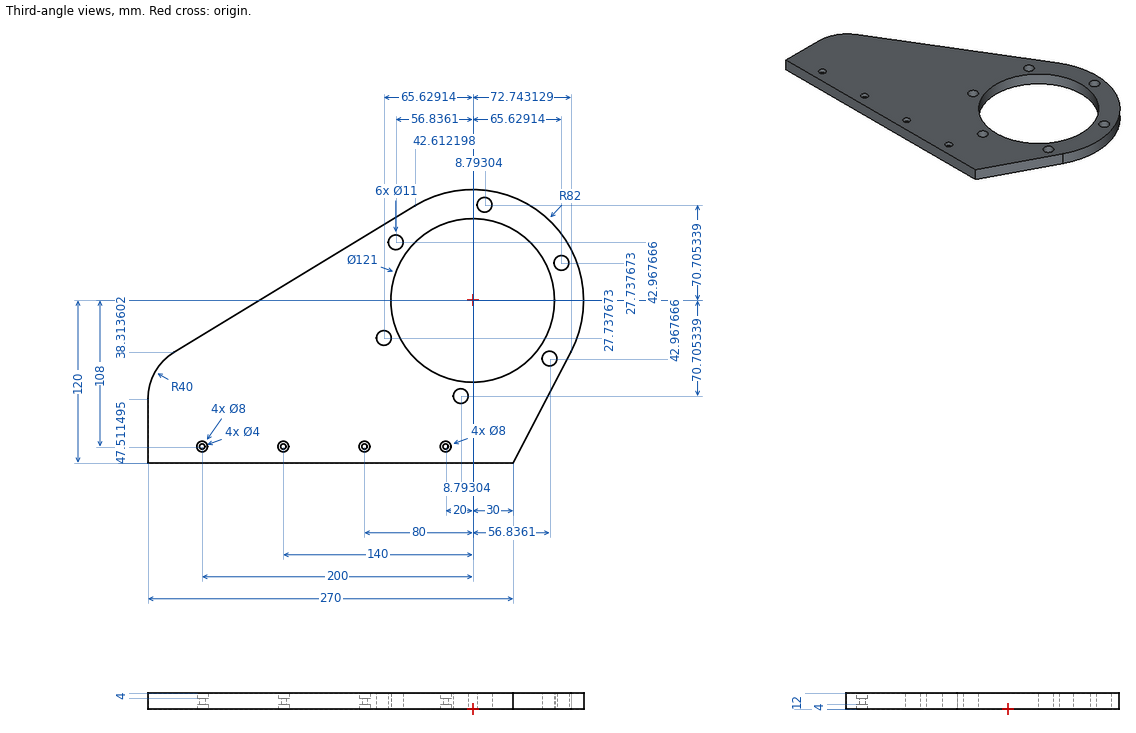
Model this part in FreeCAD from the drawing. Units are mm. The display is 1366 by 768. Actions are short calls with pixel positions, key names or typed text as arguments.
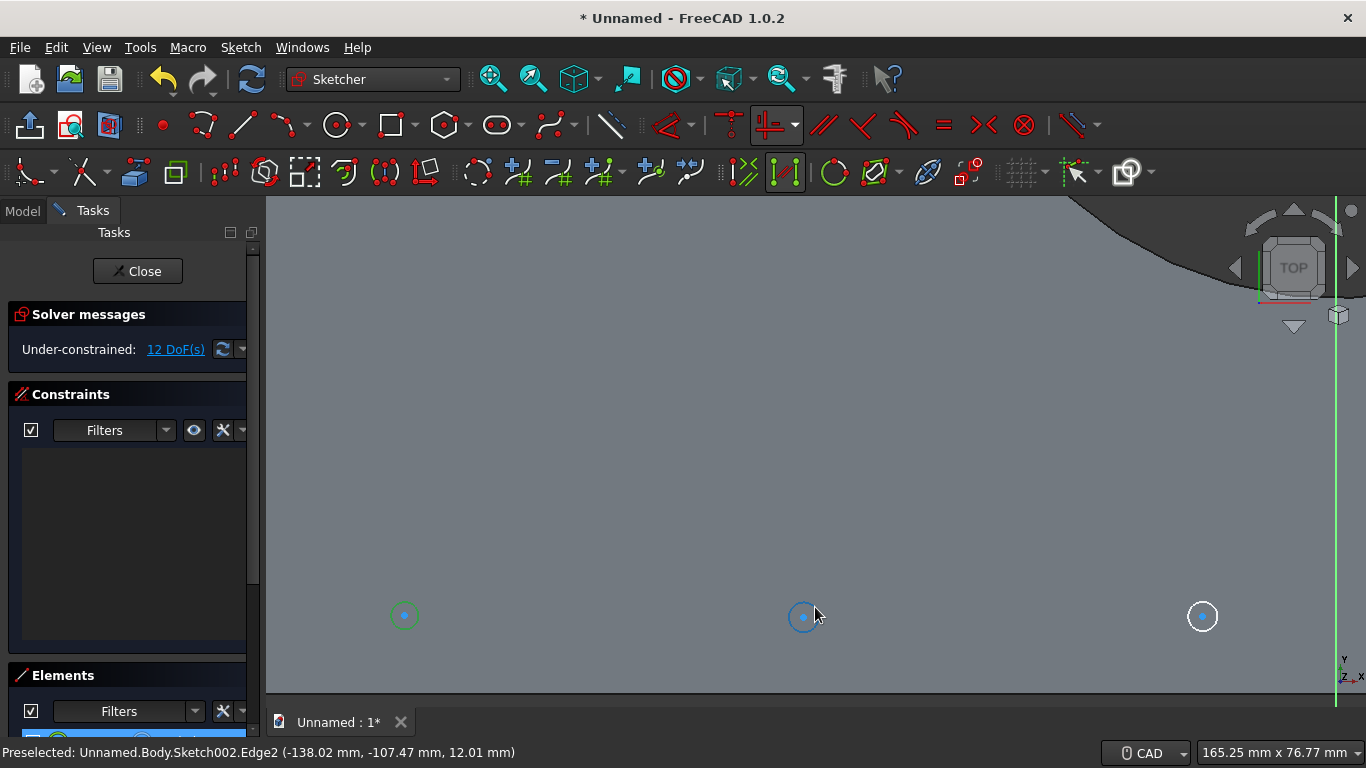
click(814, 607)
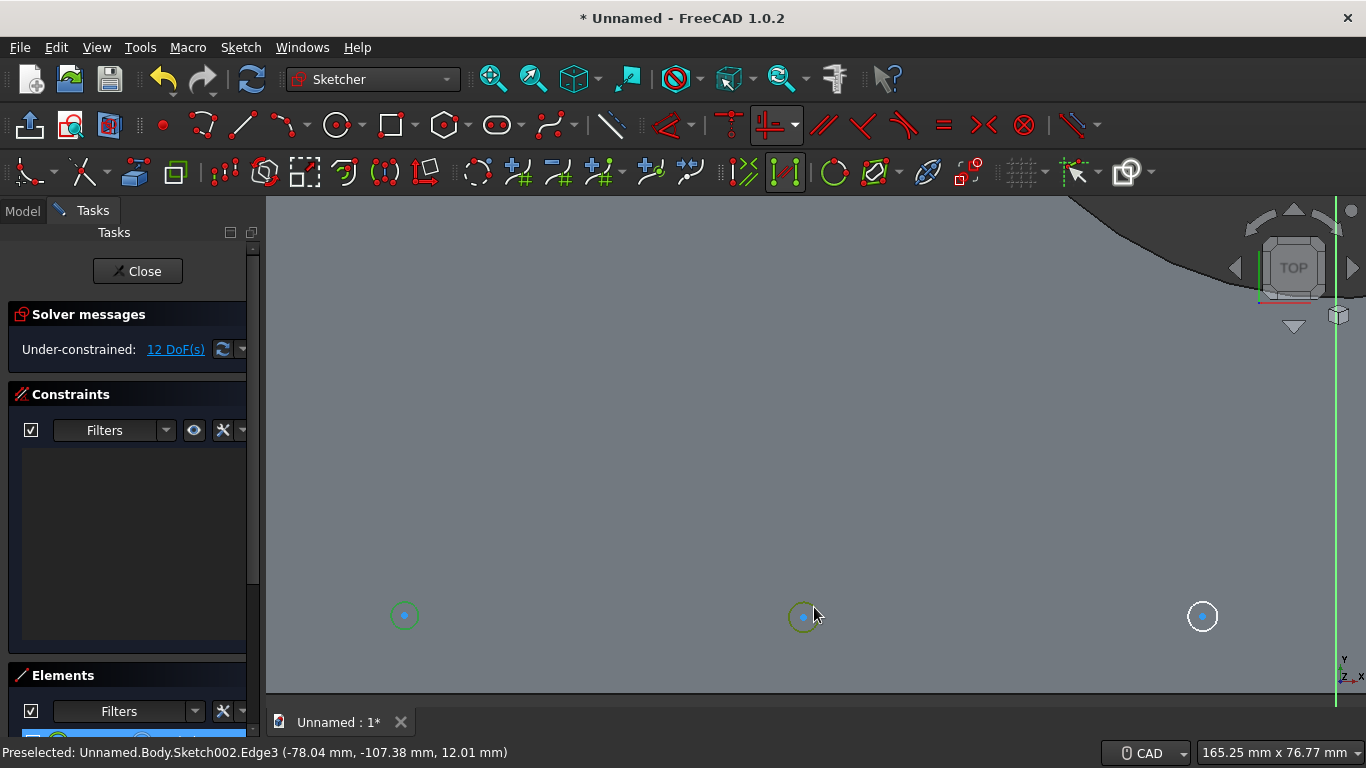
click(1193, 606)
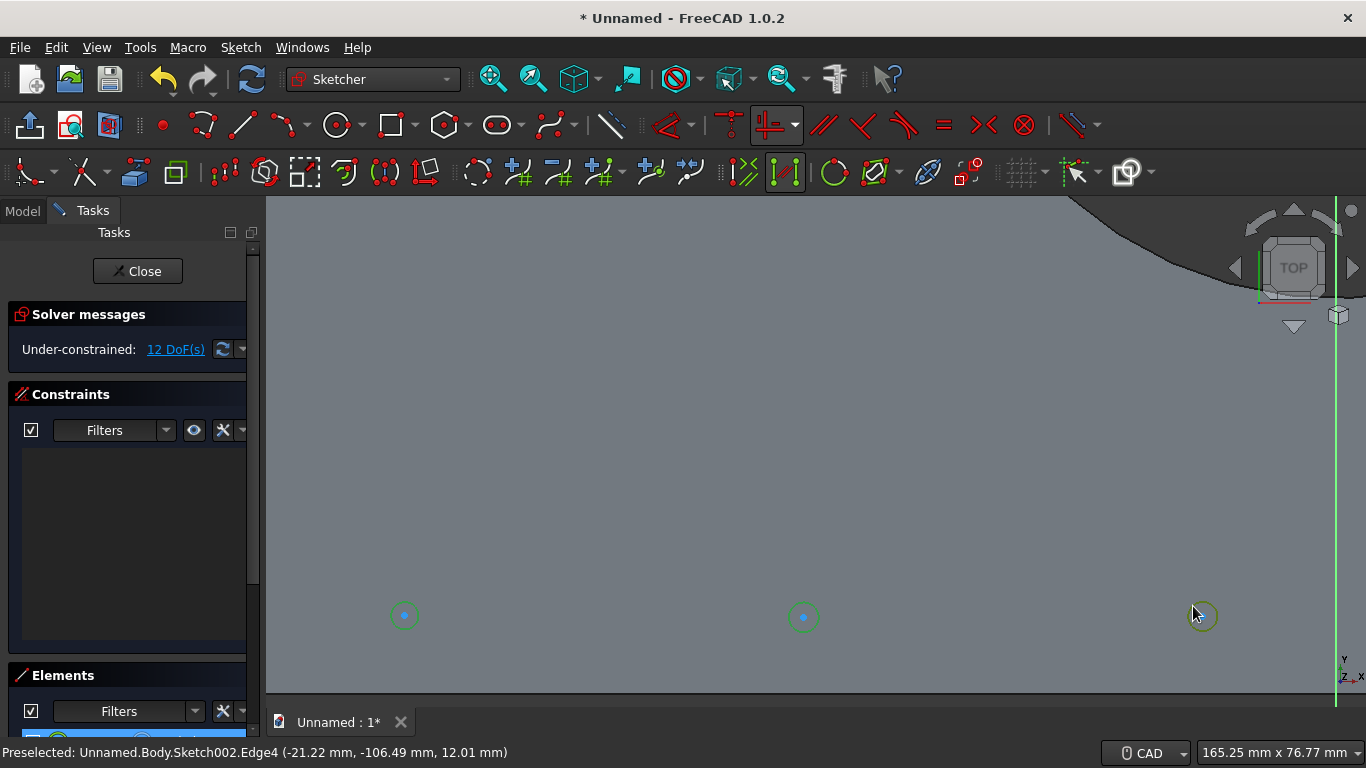
click(944, 126)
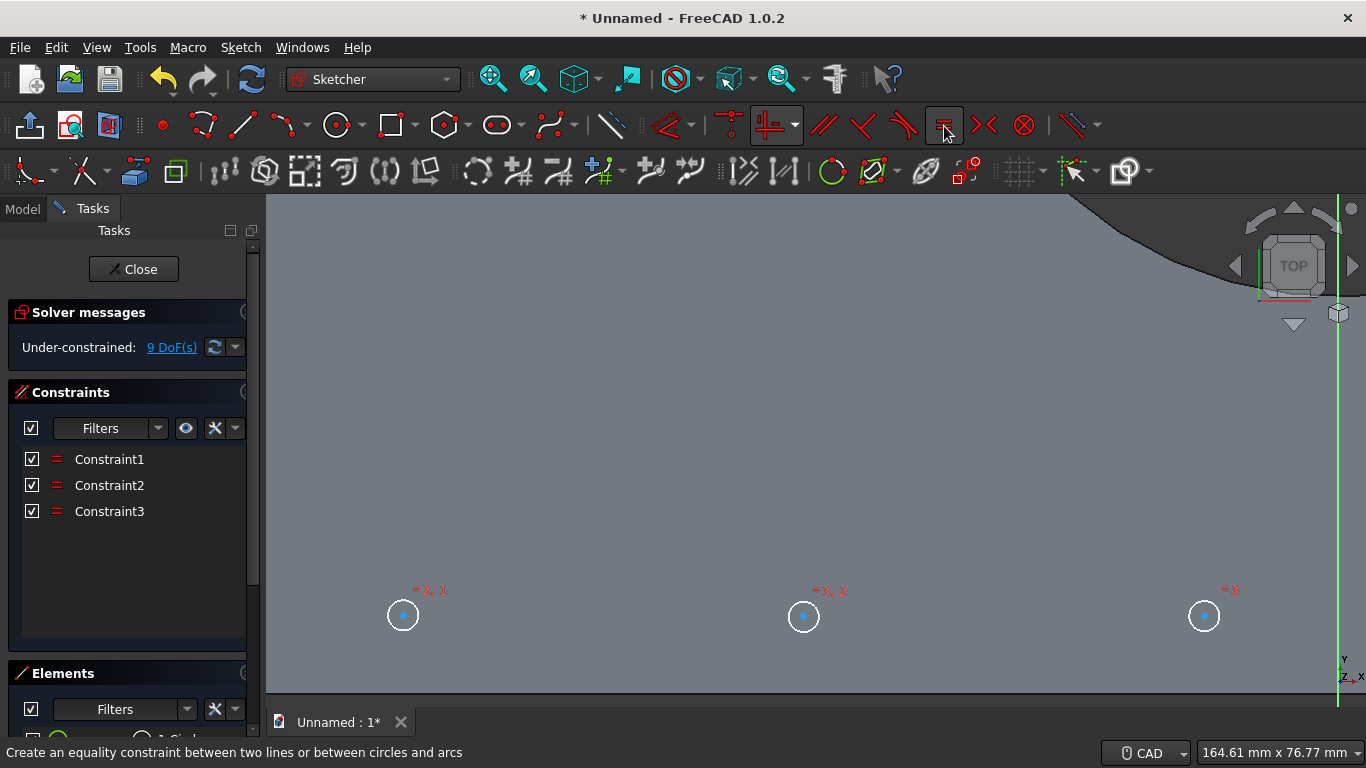
scroll(816, 606, down, 4)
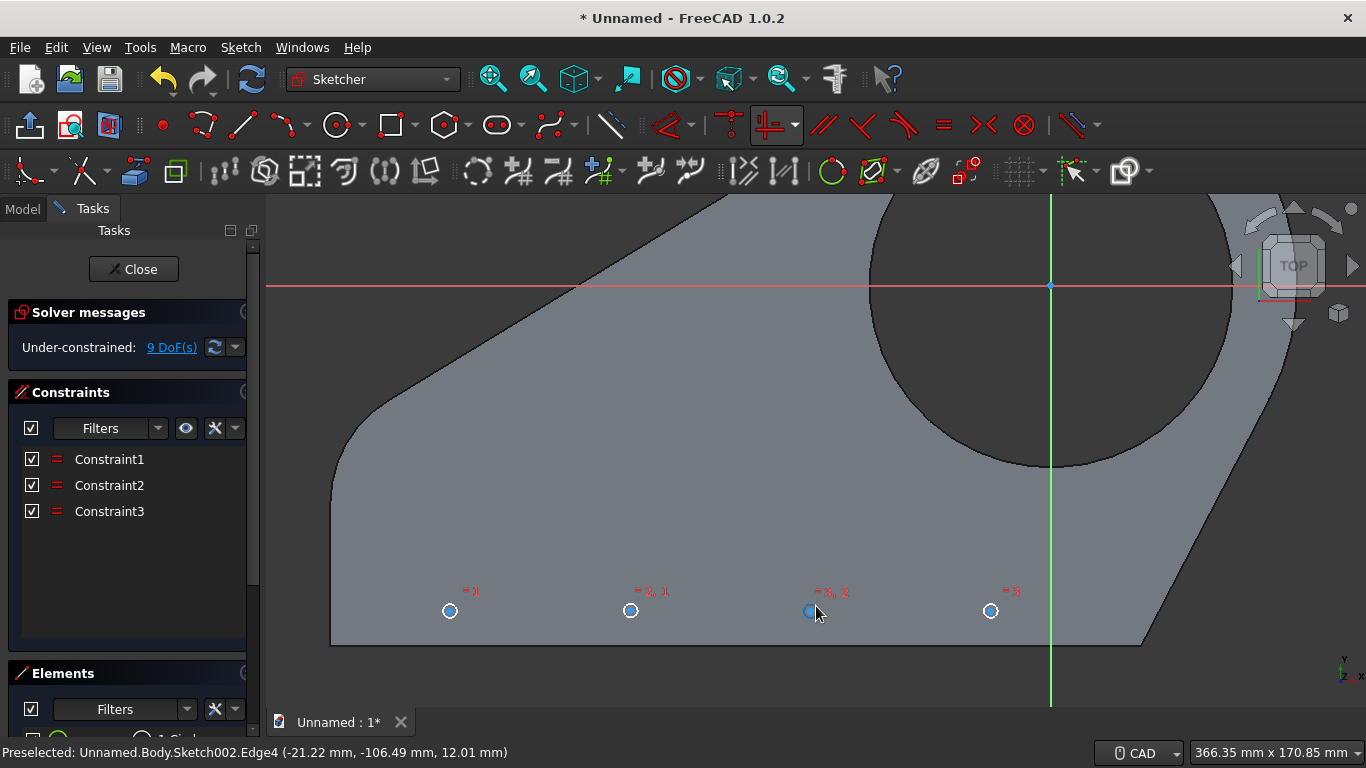
click(450, 611)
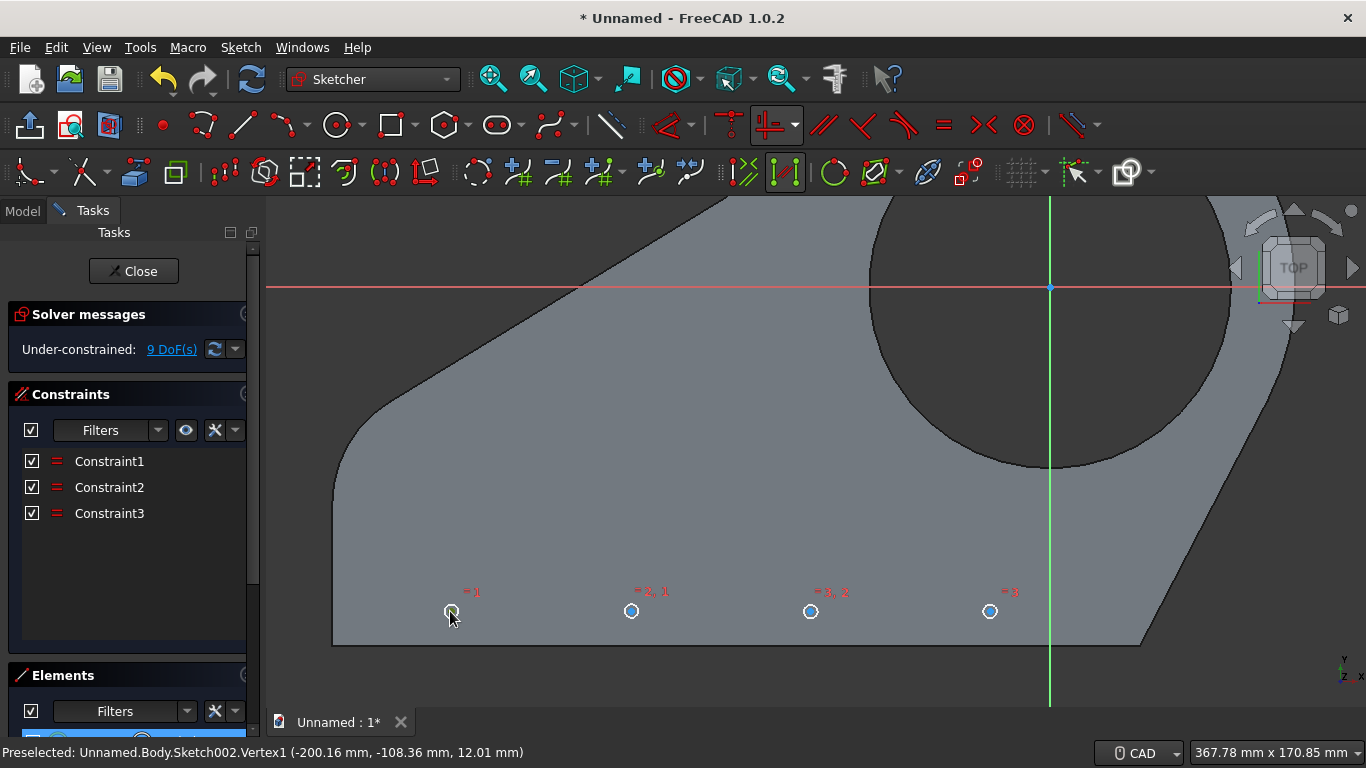
click(632, 611)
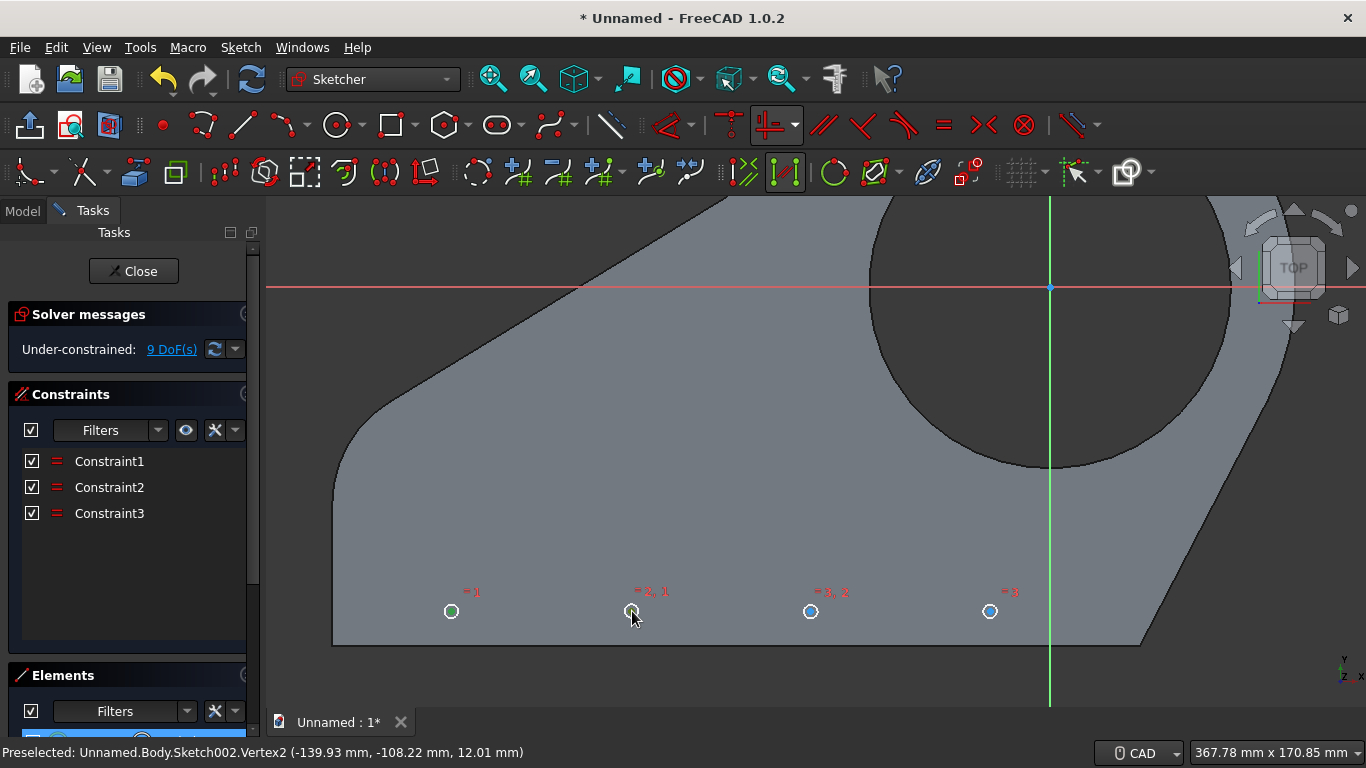
click(798, 126)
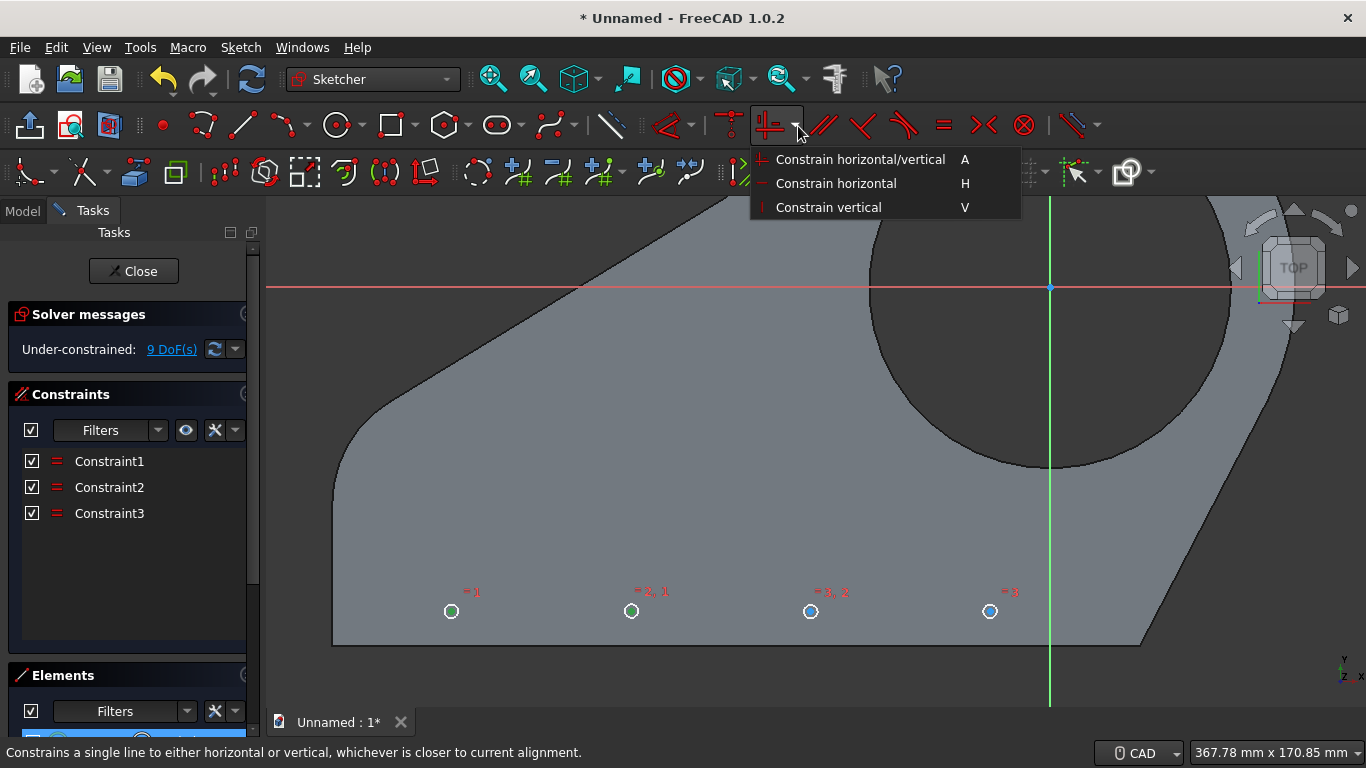
click(886, 183)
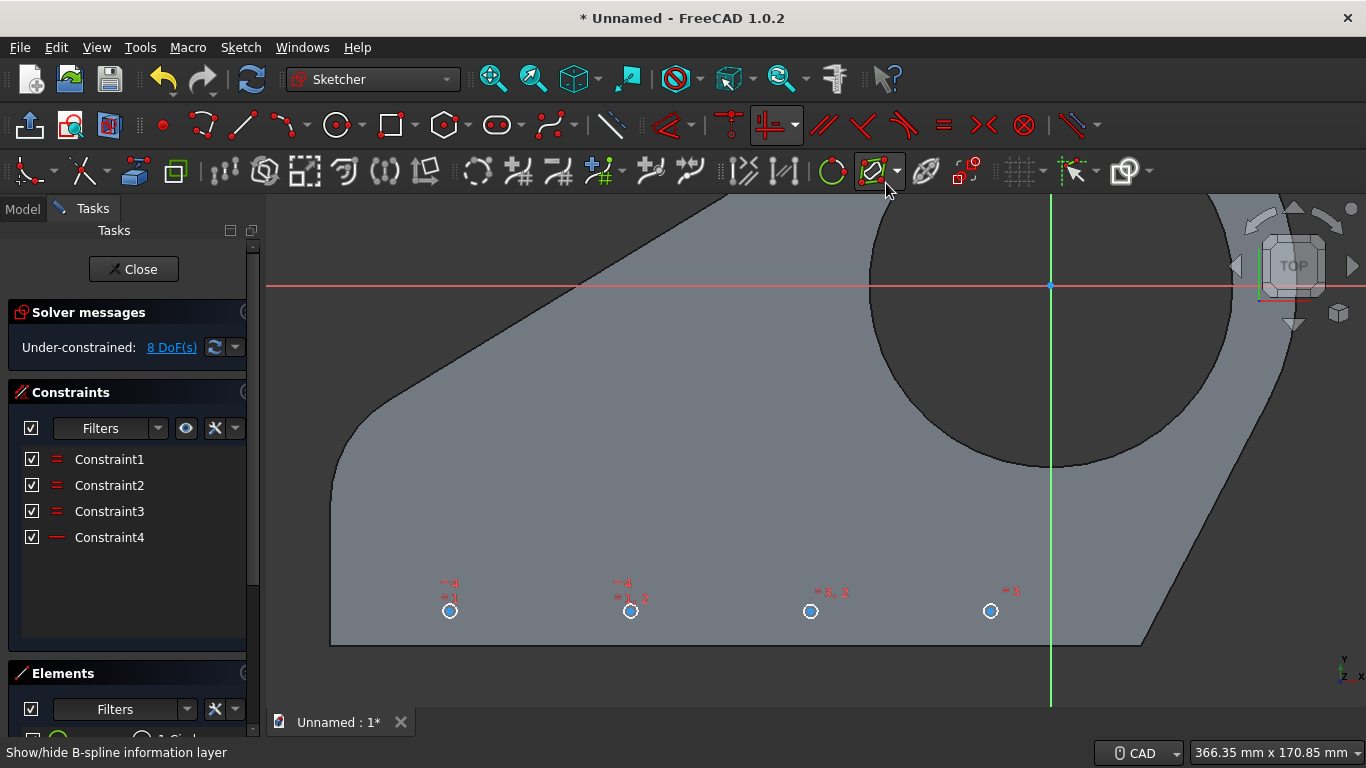
click(631, 611)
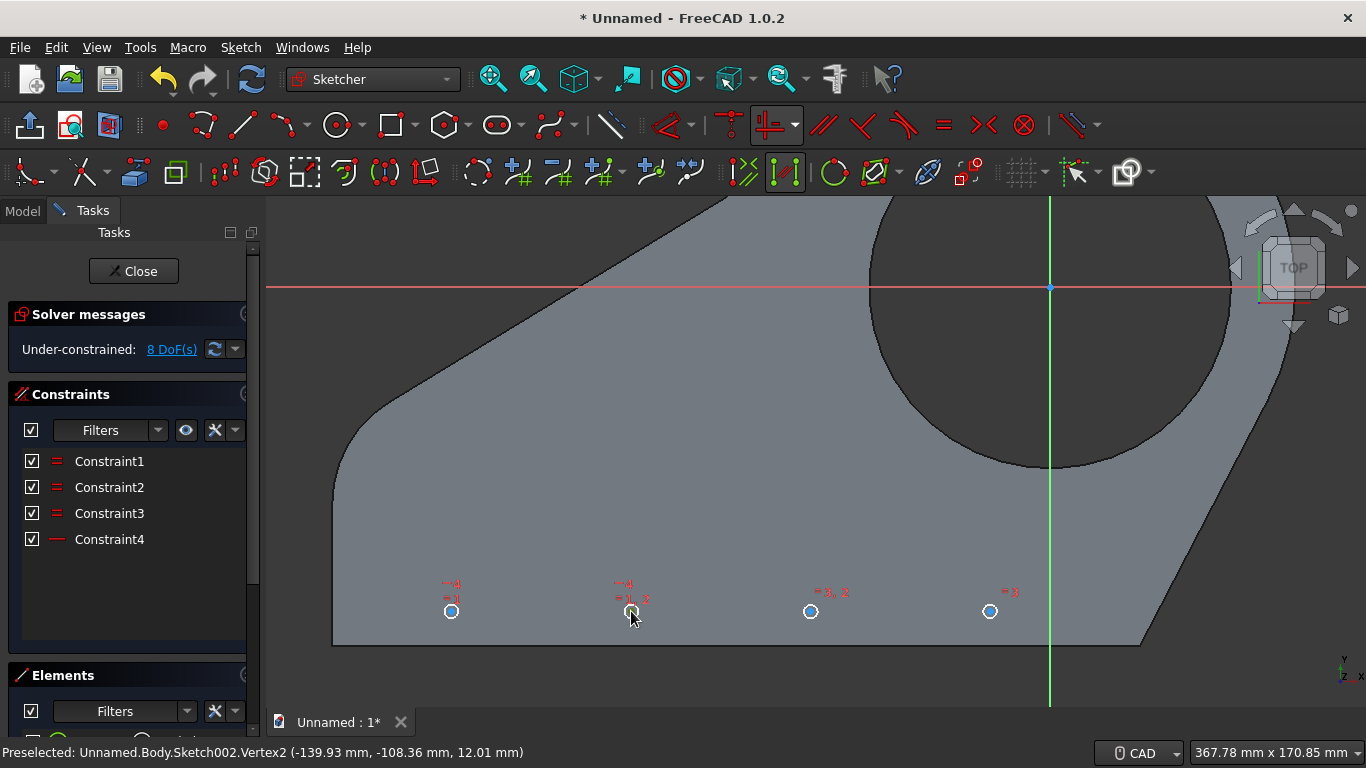
click(811, 612)